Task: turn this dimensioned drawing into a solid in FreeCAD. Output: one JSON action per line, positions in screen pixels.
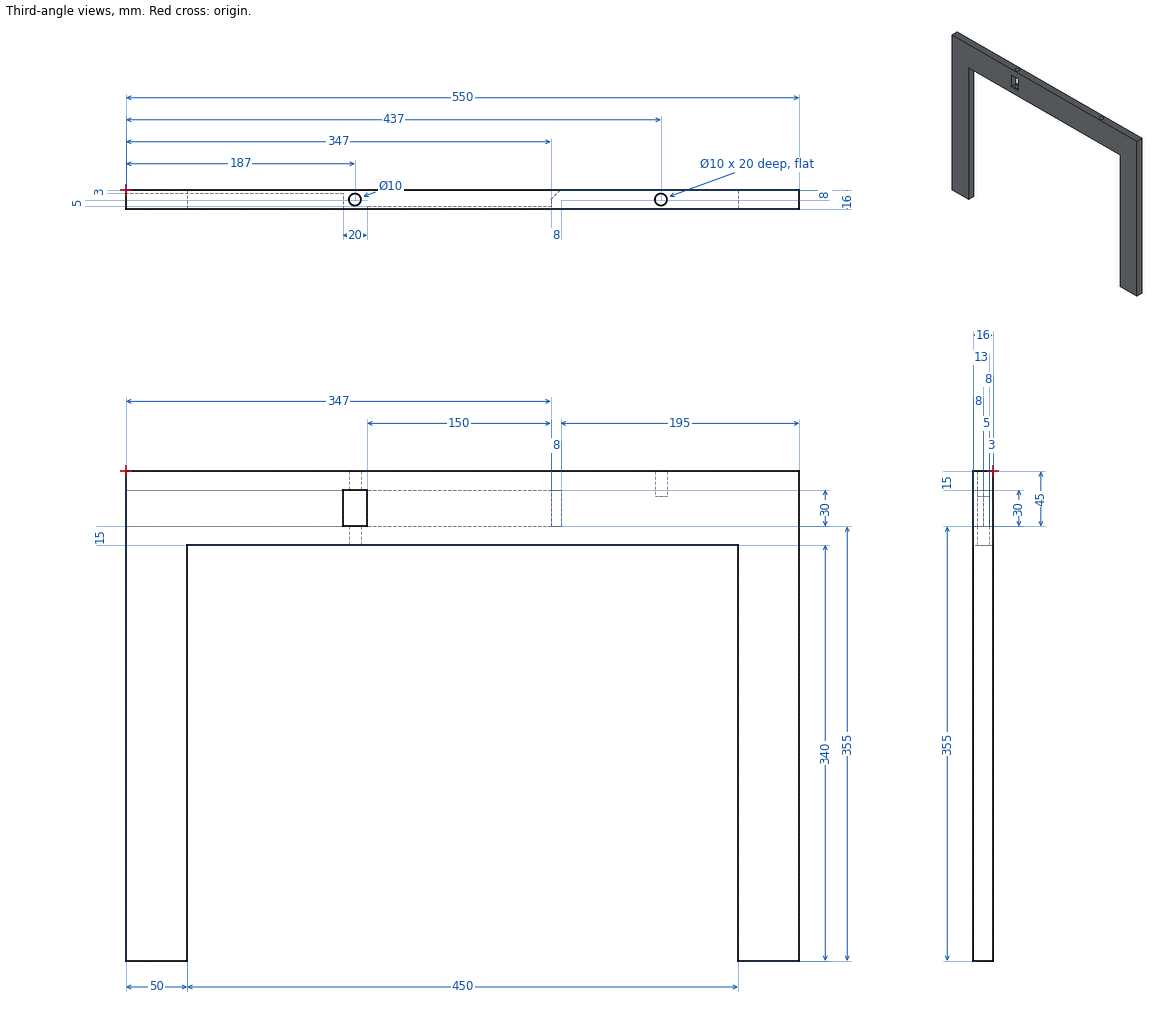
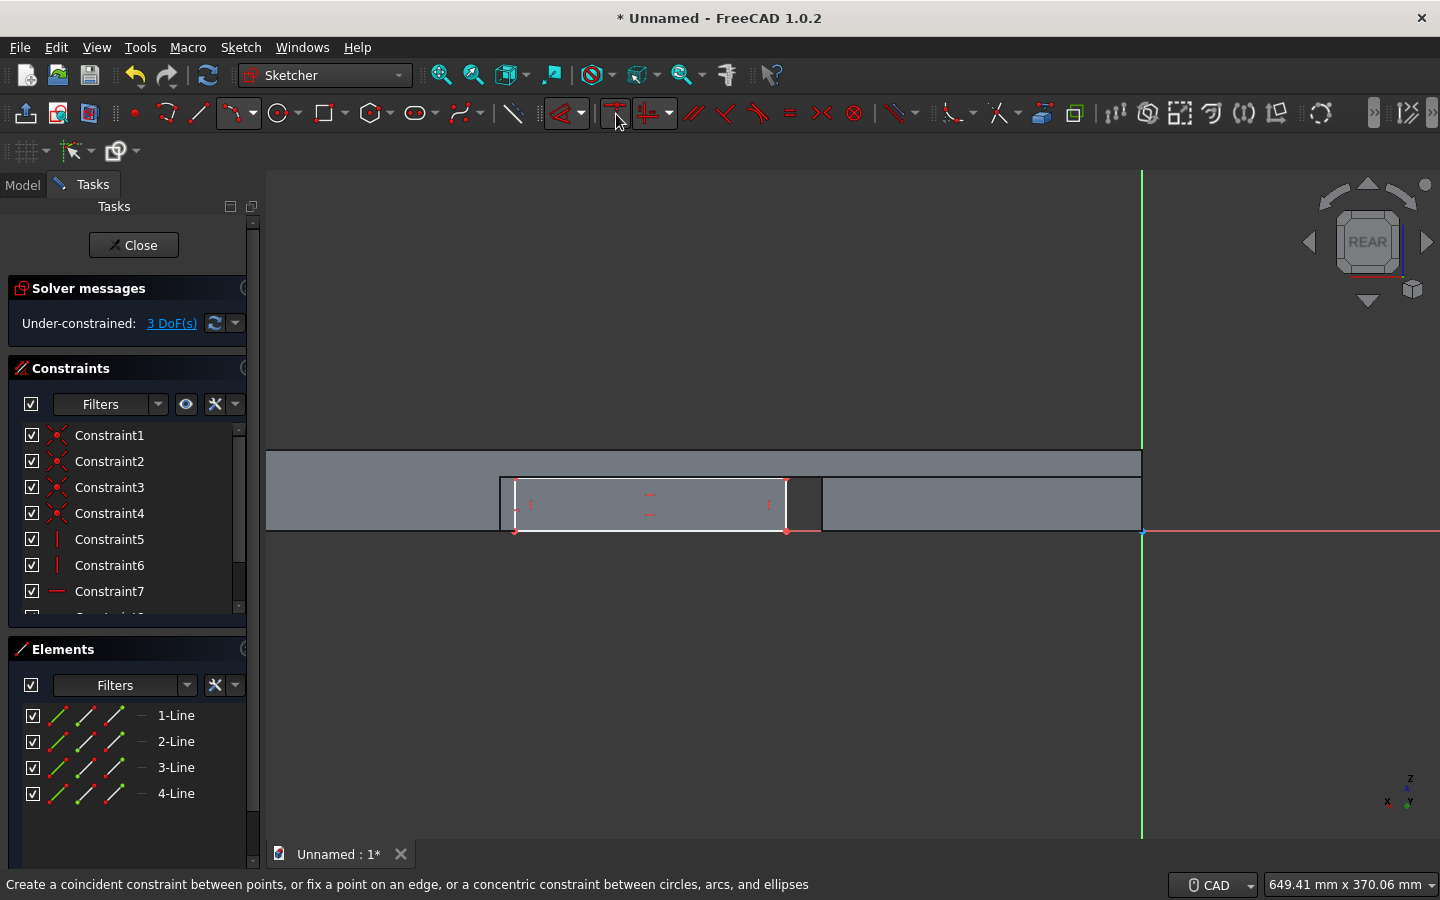
{"action": "left_click", "coordinate": [515, 494]}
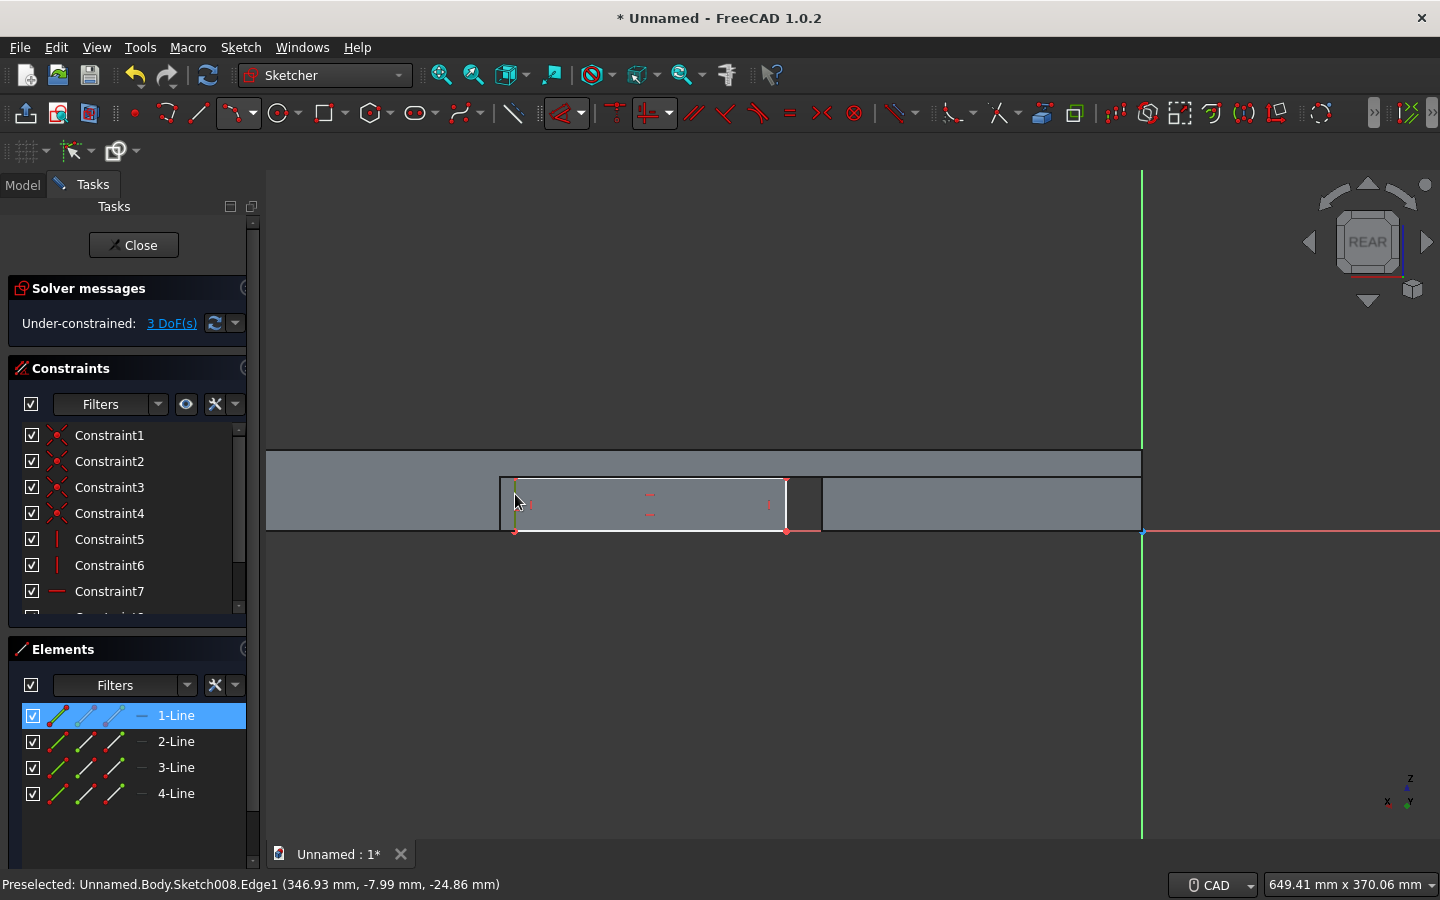
{"action": "key", "text": "i"}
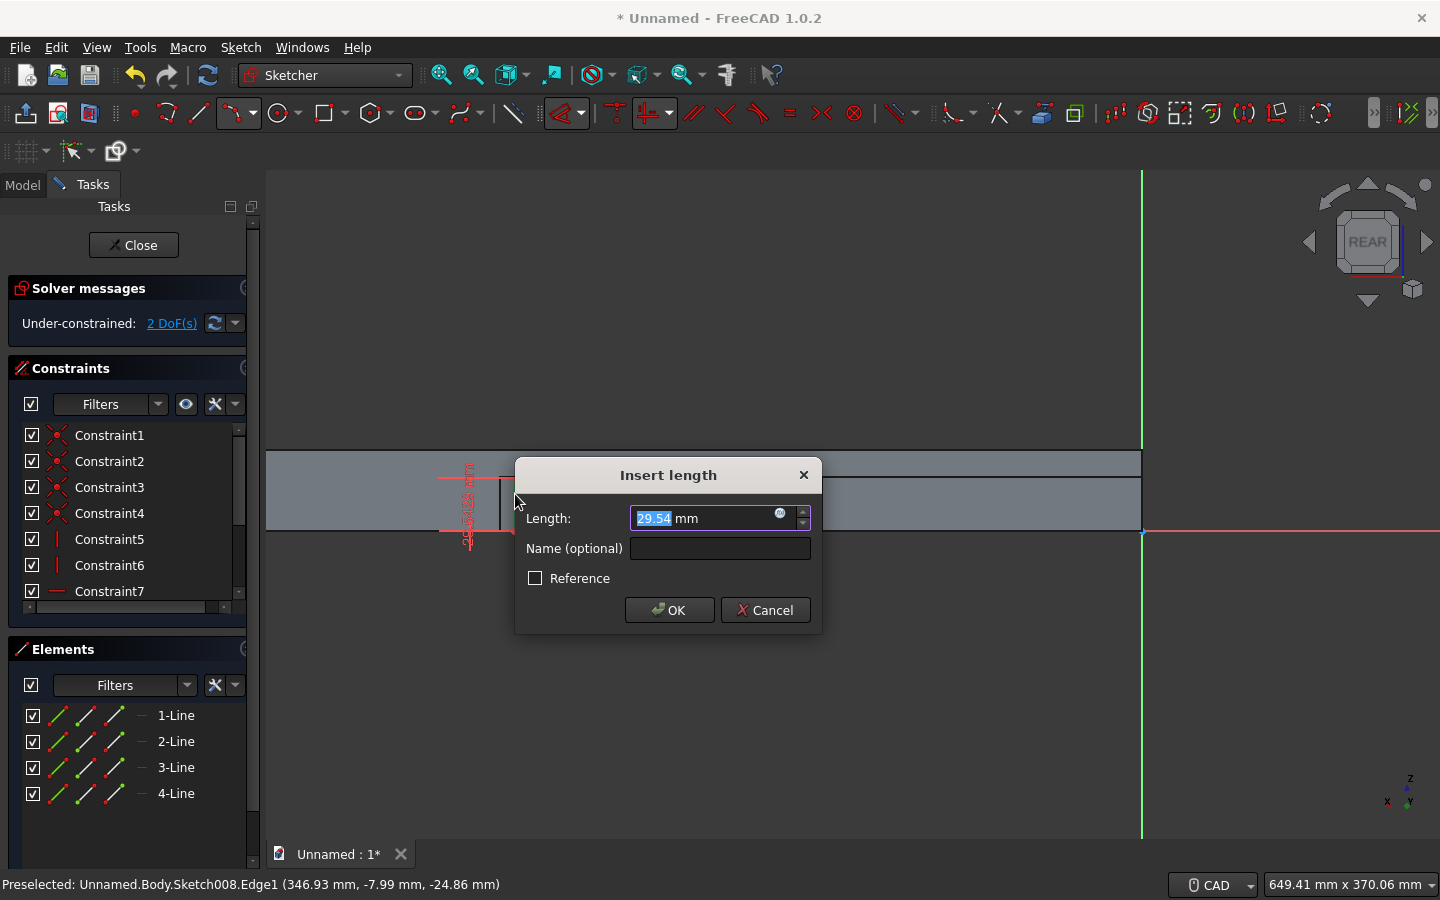
{"action": "type", "text": "30"}
{"action": "key", "text": "Return"}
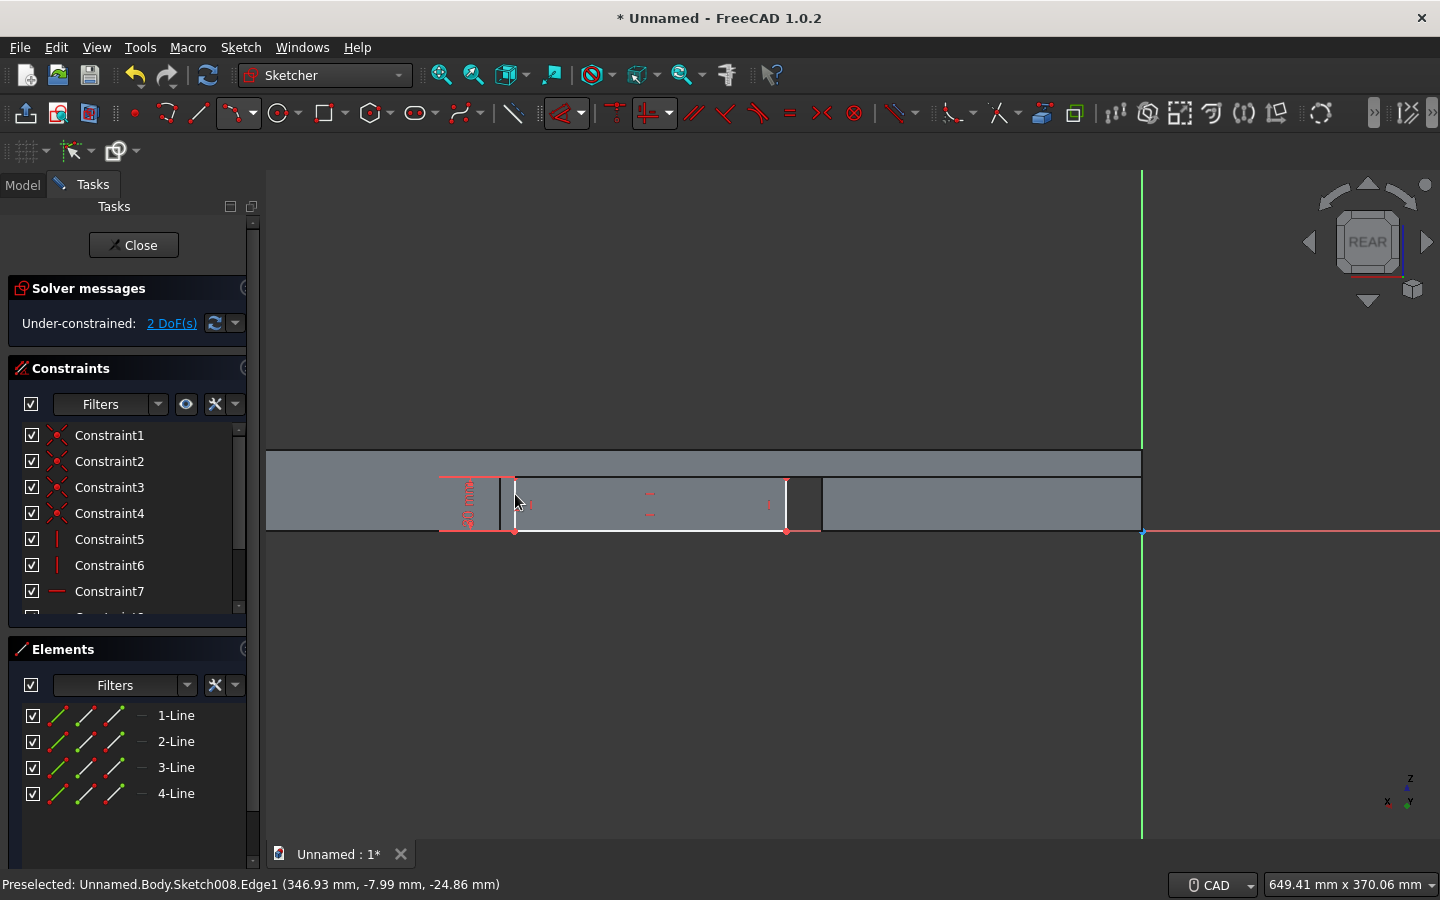
{"action": "left_click", "coordinate": [596, 531]}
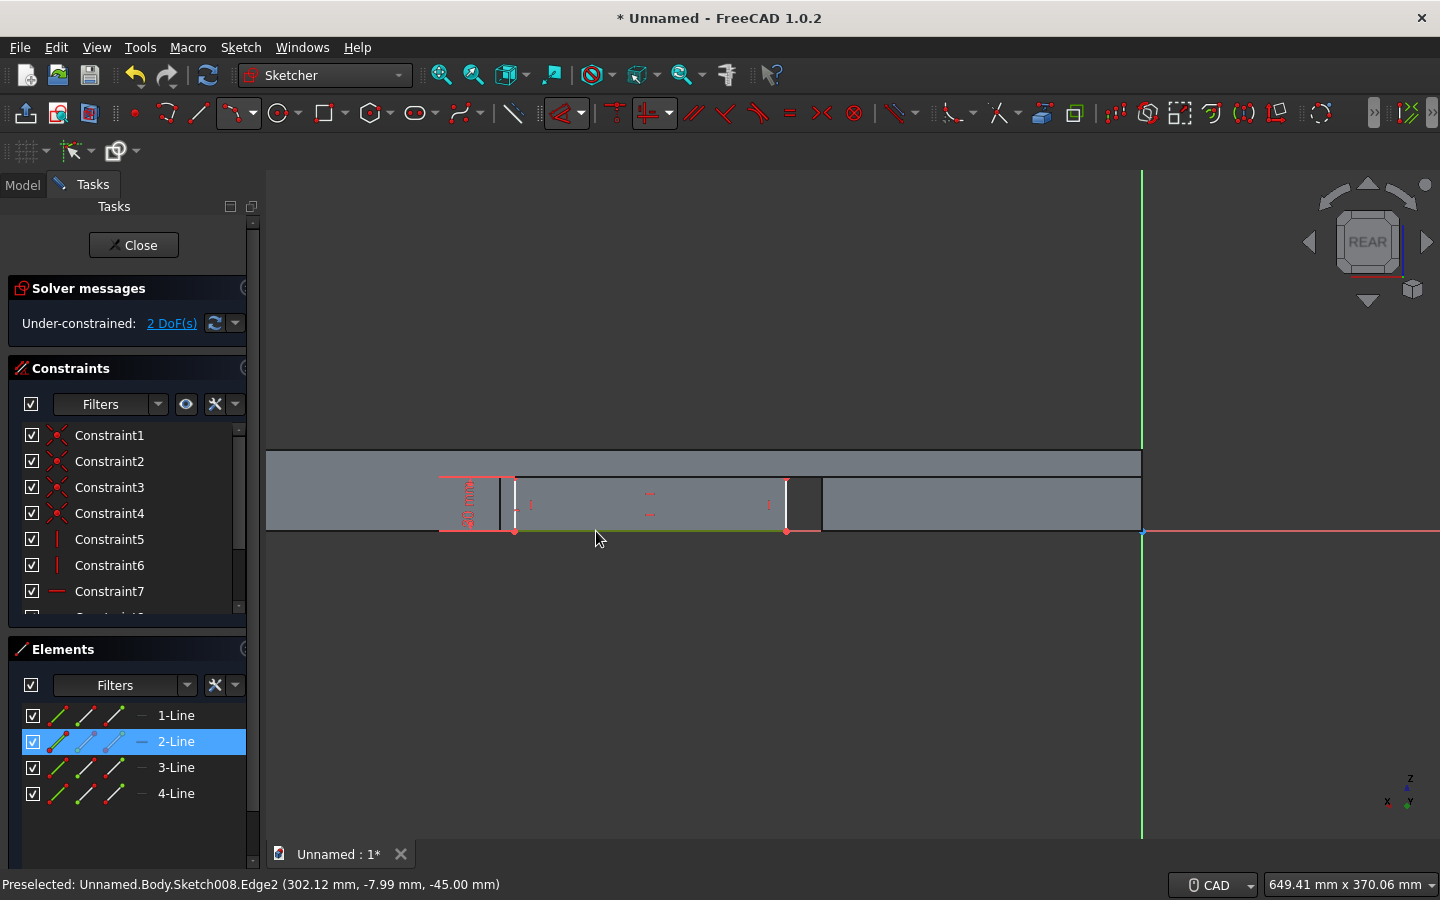
{"action": "left_click", "coordinate": [584, 114]}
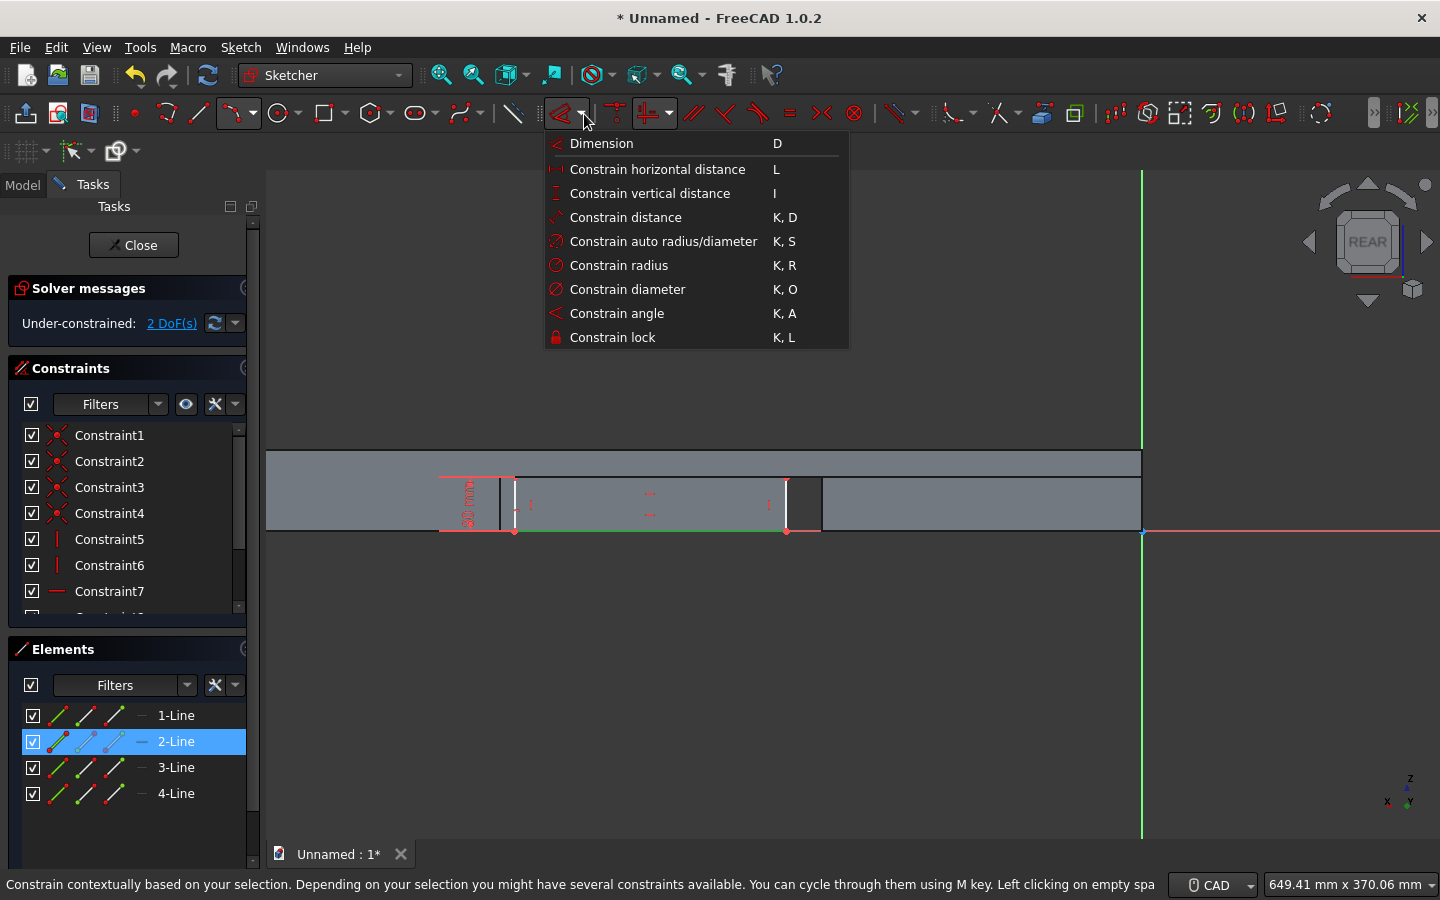
{"action": "left_click", "coordinate": [697, 169]}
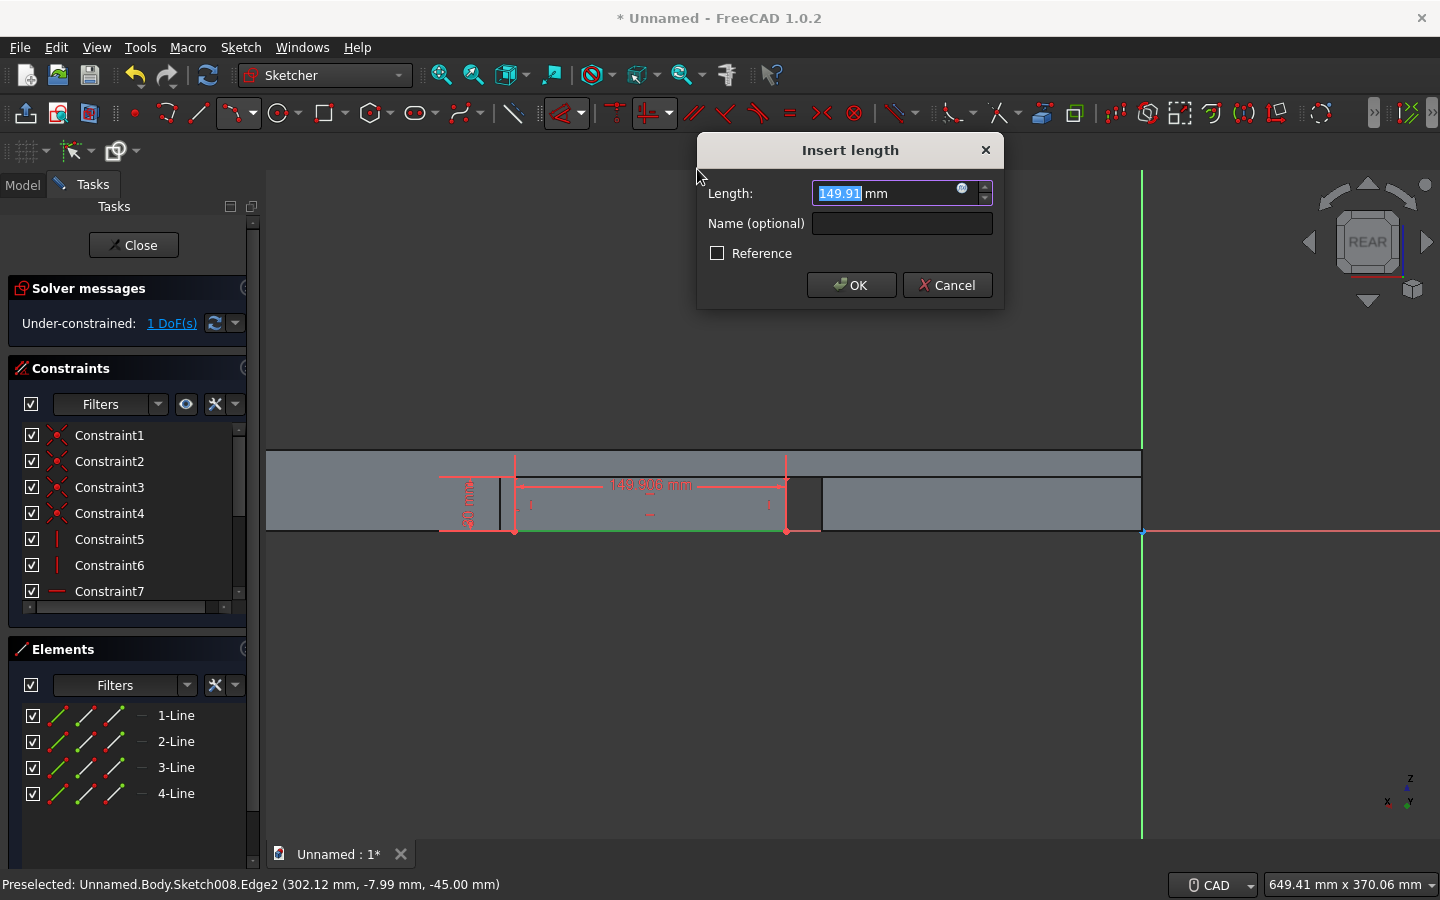
{"action": "type", "text": "150"}
{"action": "key", "text": "Return"}